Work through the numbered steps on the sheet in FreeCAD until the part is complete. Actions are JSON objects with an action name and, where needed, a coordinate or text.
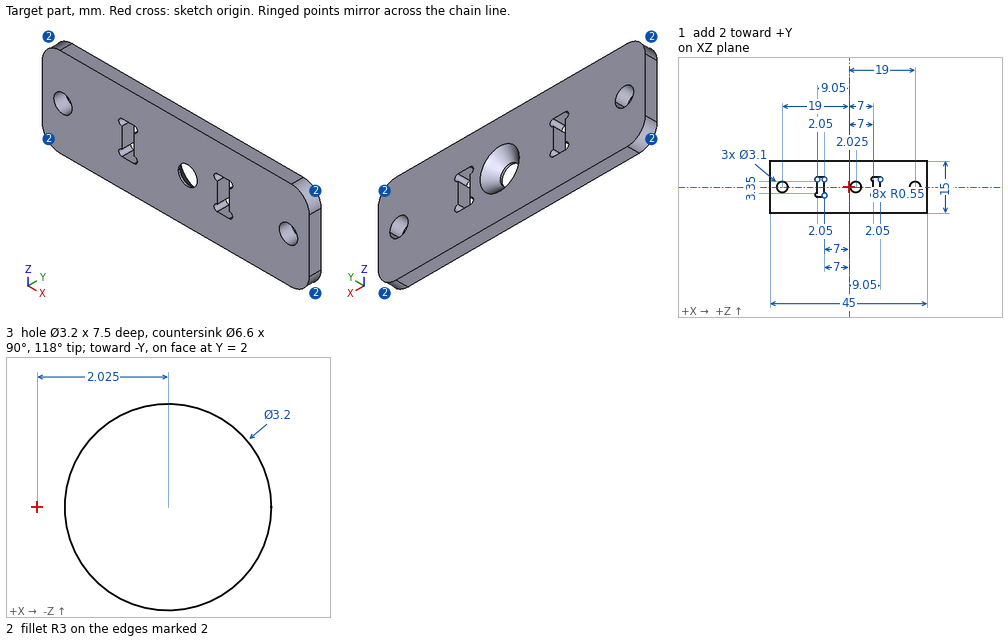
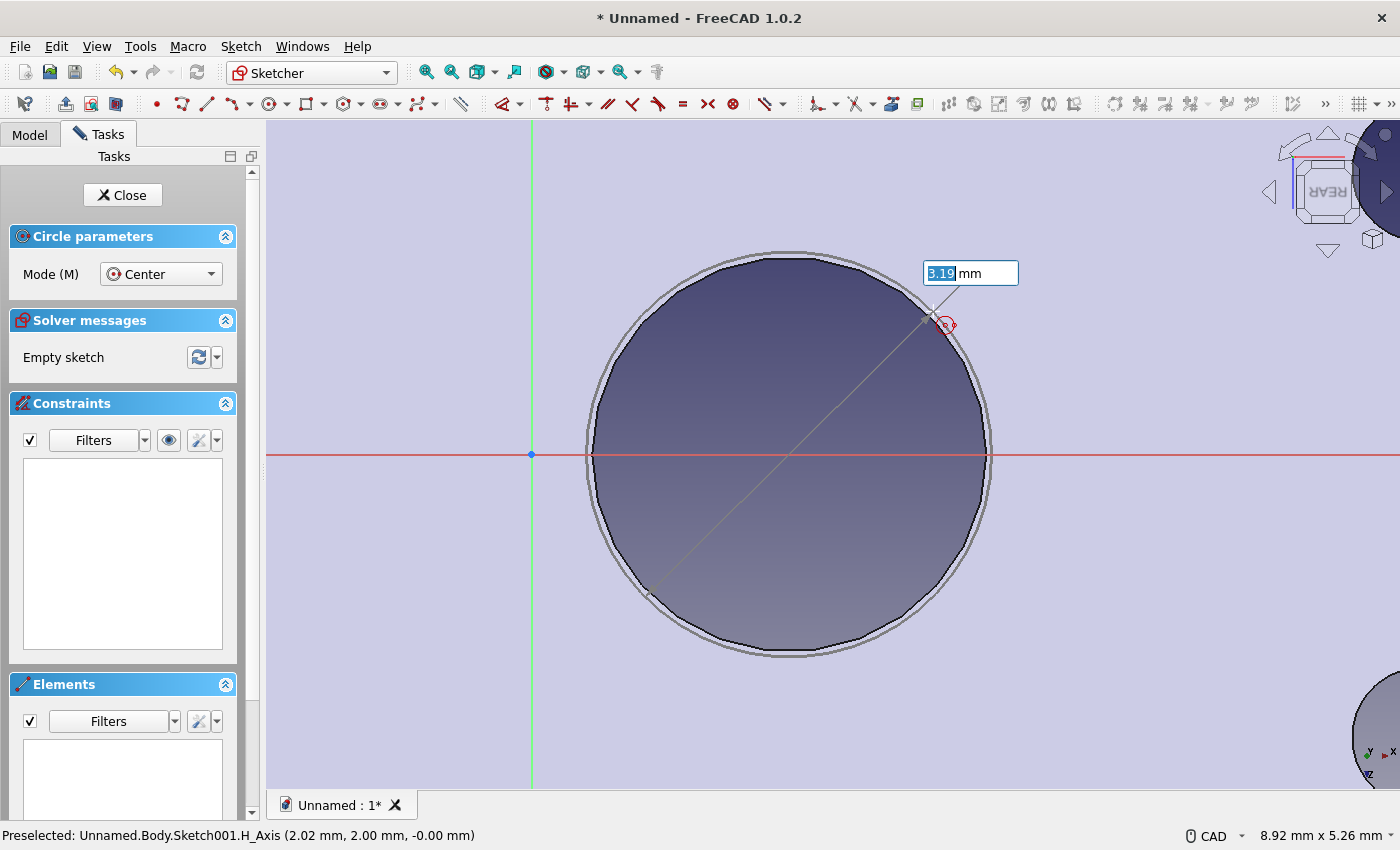
{"action": "type", "text": "3.2"}
{"action": "key", "text": "Return"}
{"action": "key", "text": "Escape"}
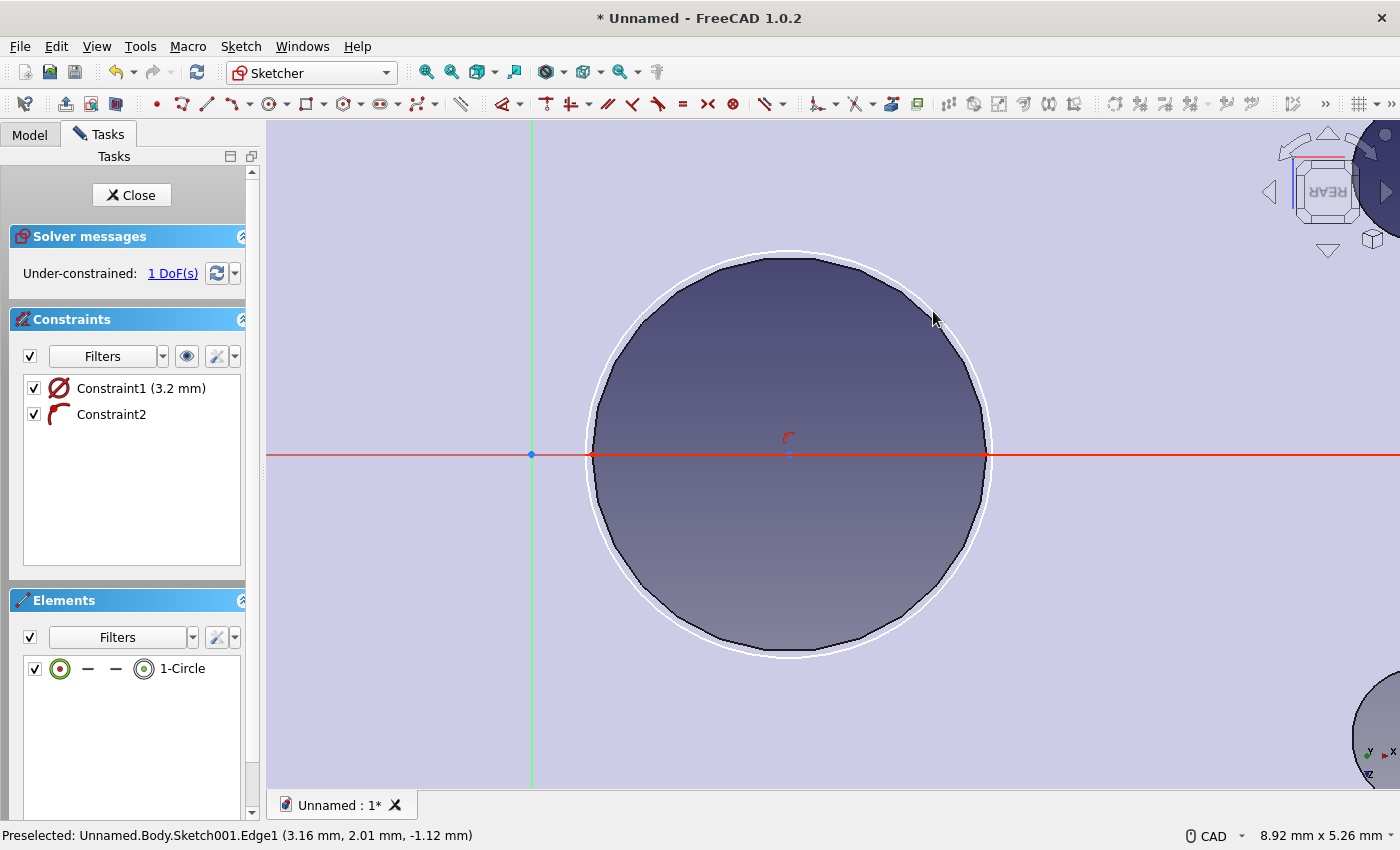
{"action": "left_click", "coordinate": [502, 104]}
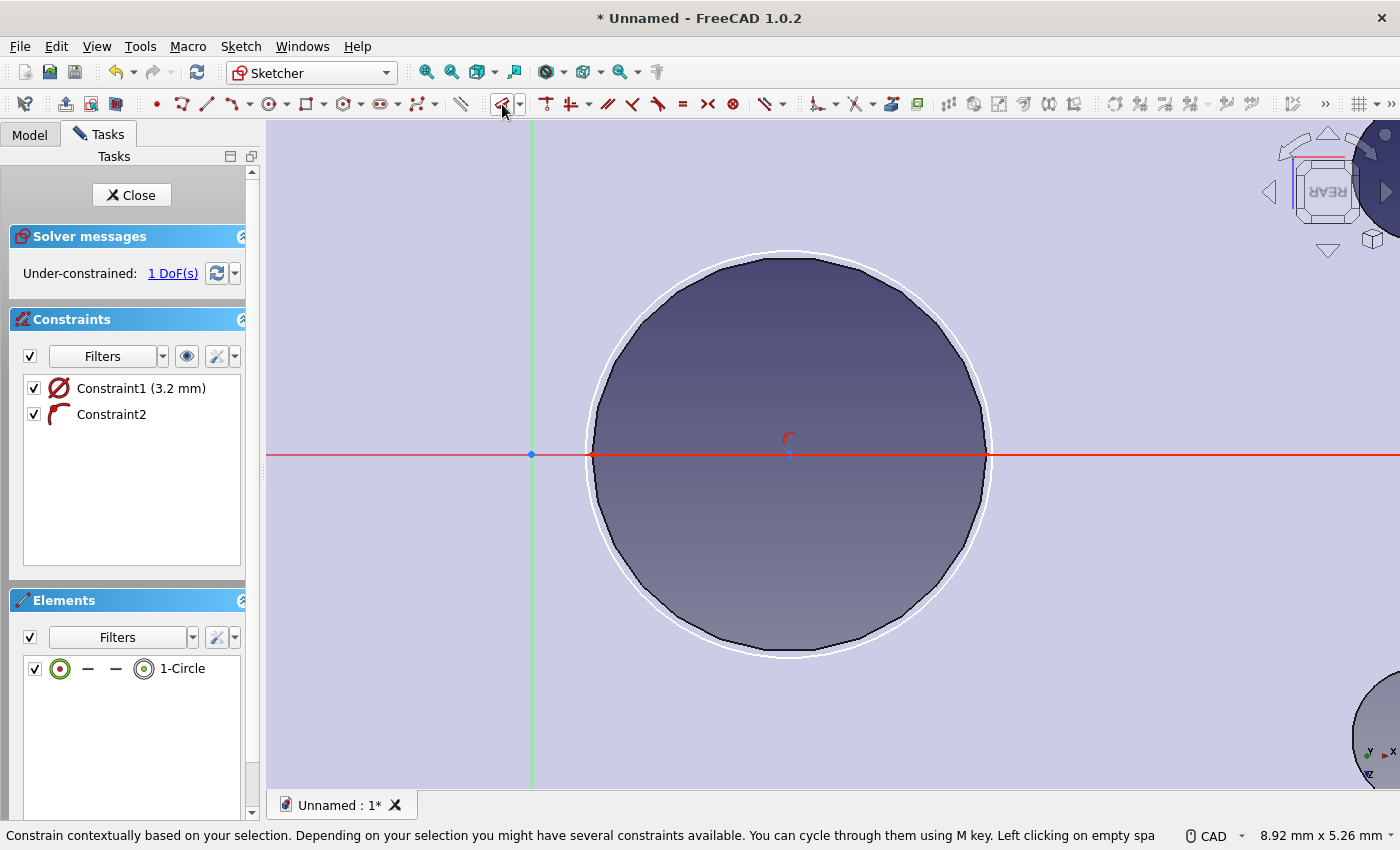
{"action": "left_click", "coordinate": [789, 454]}
{"action": "left_click", "coordinate": [660, 488]}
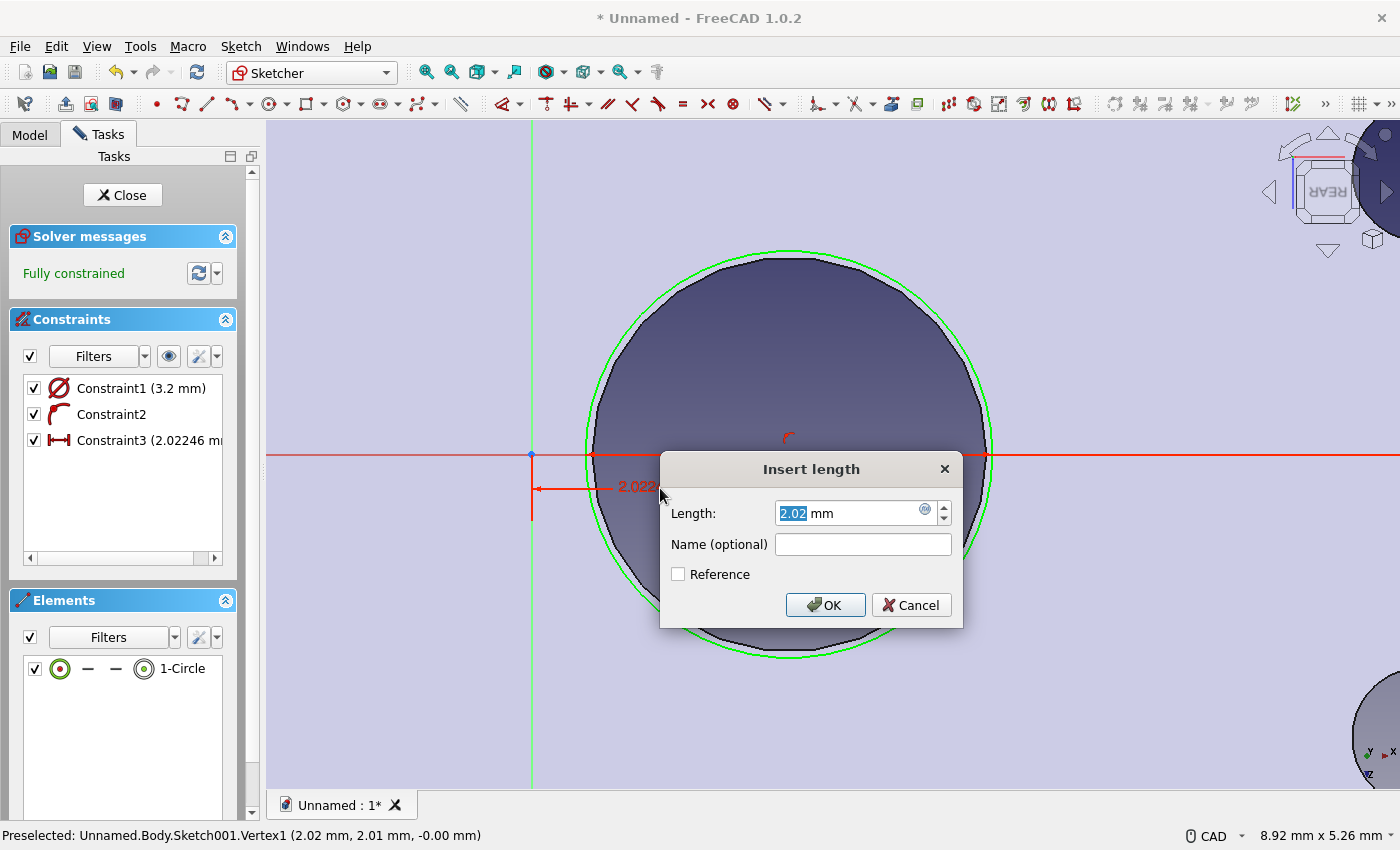
{"action": "type", "text": "2.025"}
{"action": "key", "text": "Return"}
{"action": "key", "text": "Escape"}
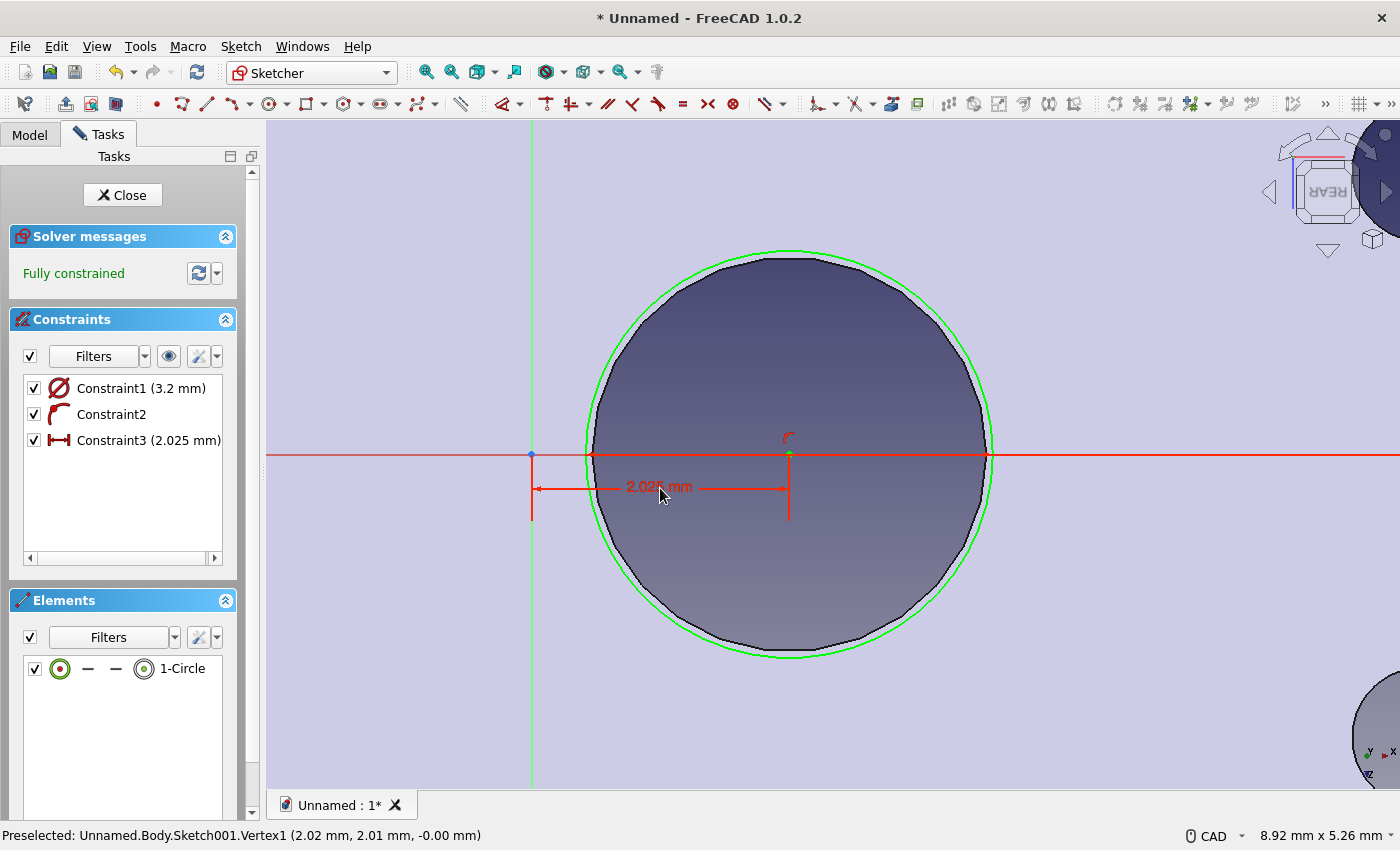
{"action": "left_click", "coordinate": [123, 195]}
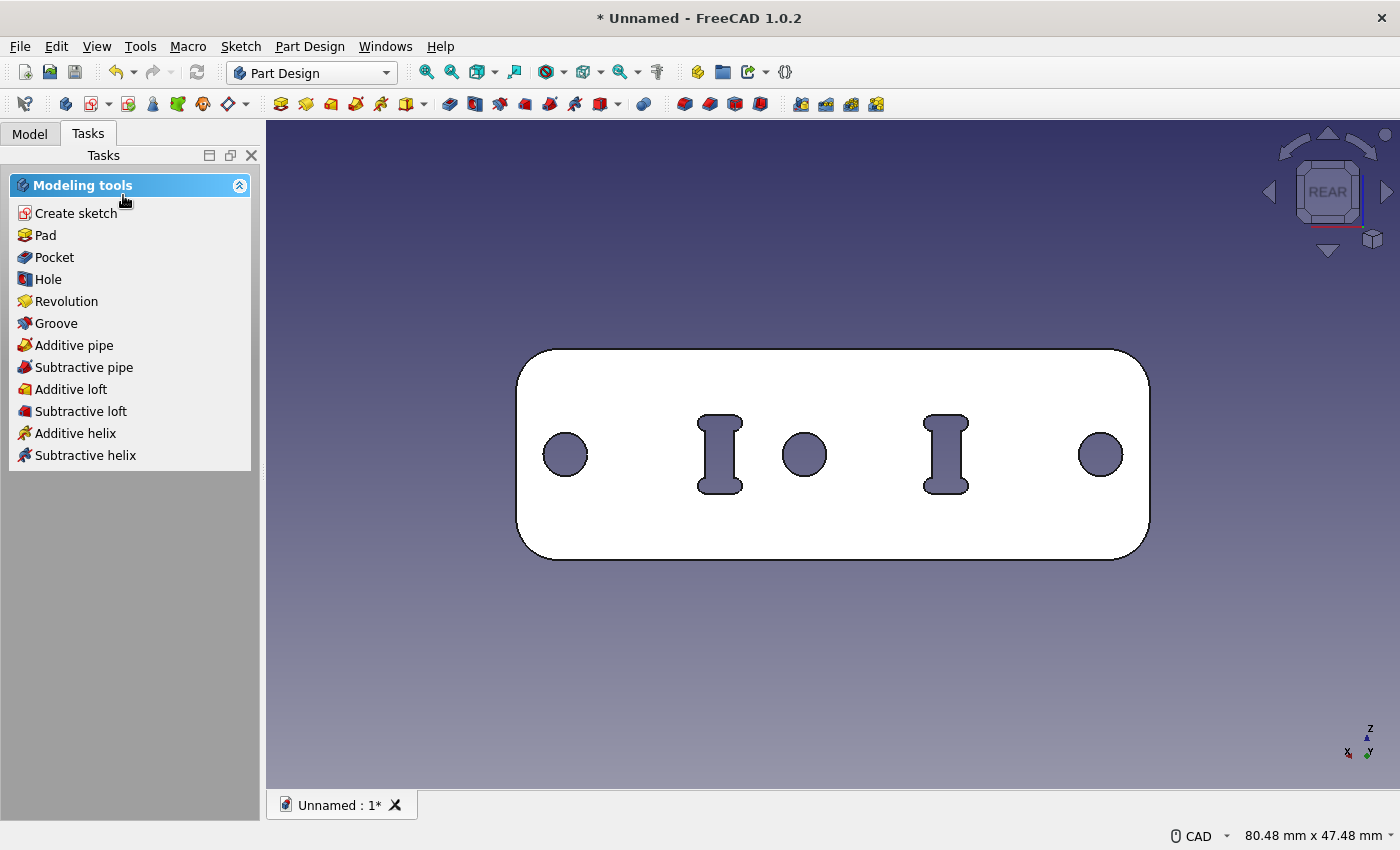
{"action": "left_click", "coordinate": [475, 104]}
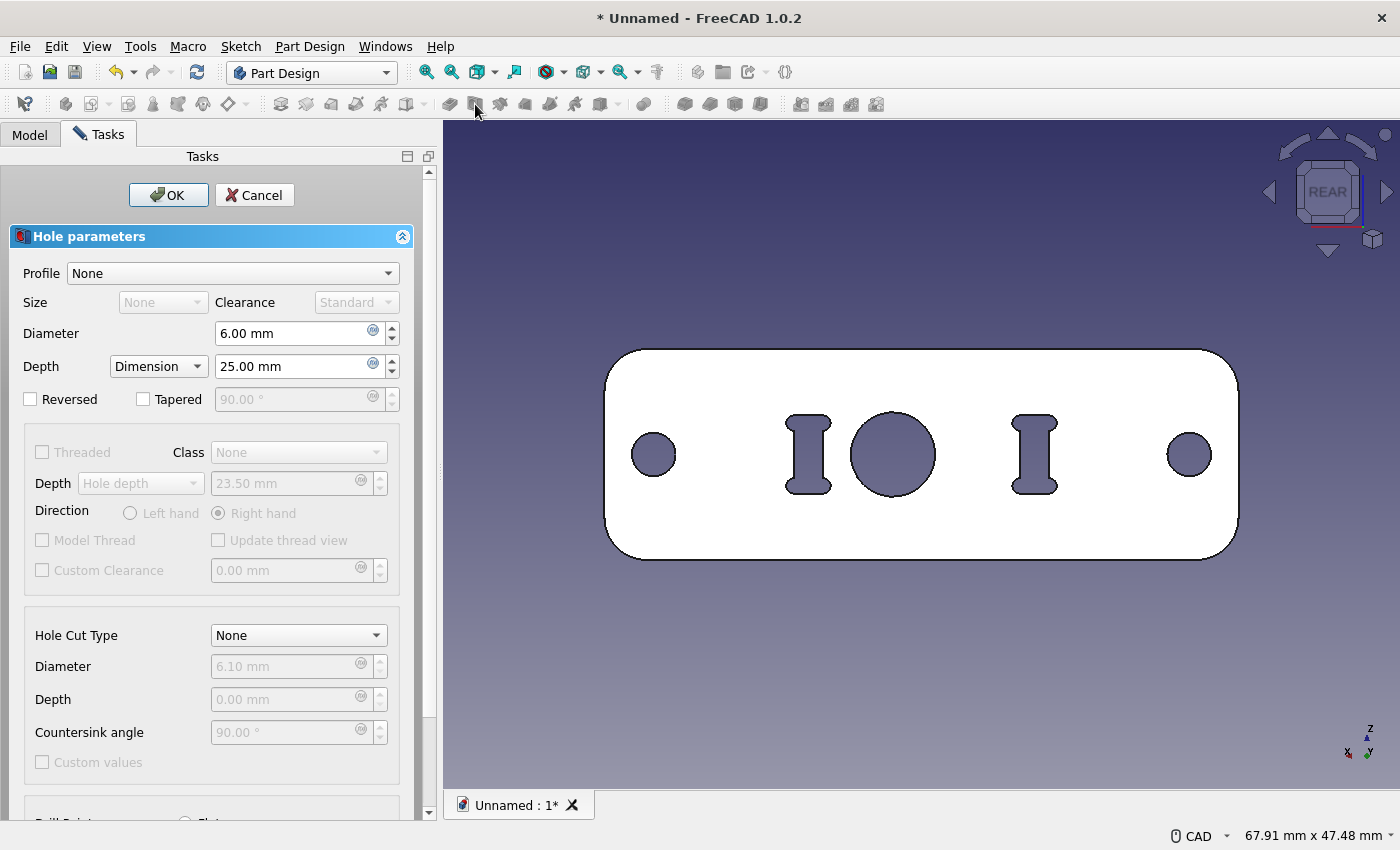
{"action": "triple_click", "coordinate": [300, 334]}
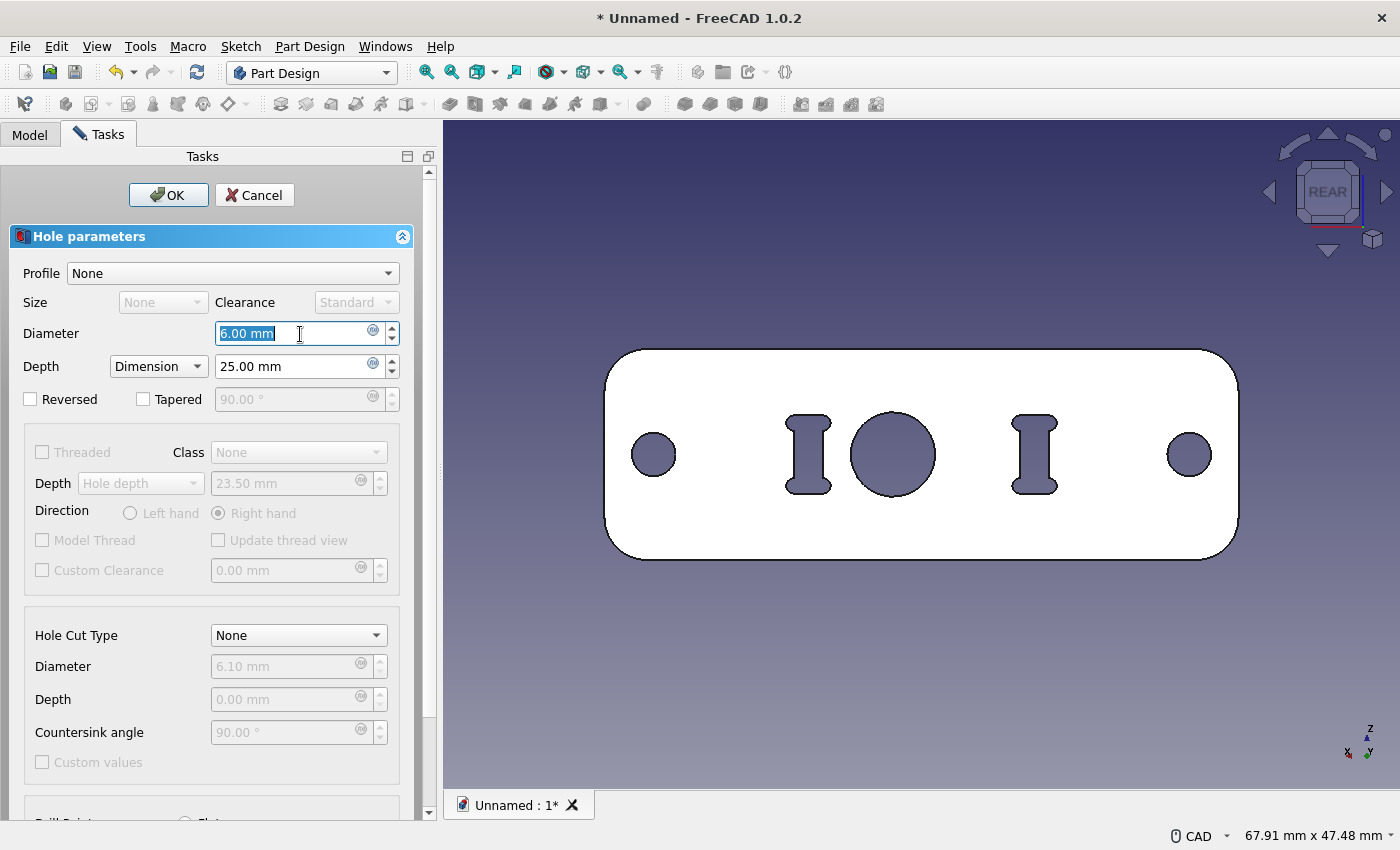
{"action": "type", "text": "3.2"}
{"action": "key", "text": "Tab"}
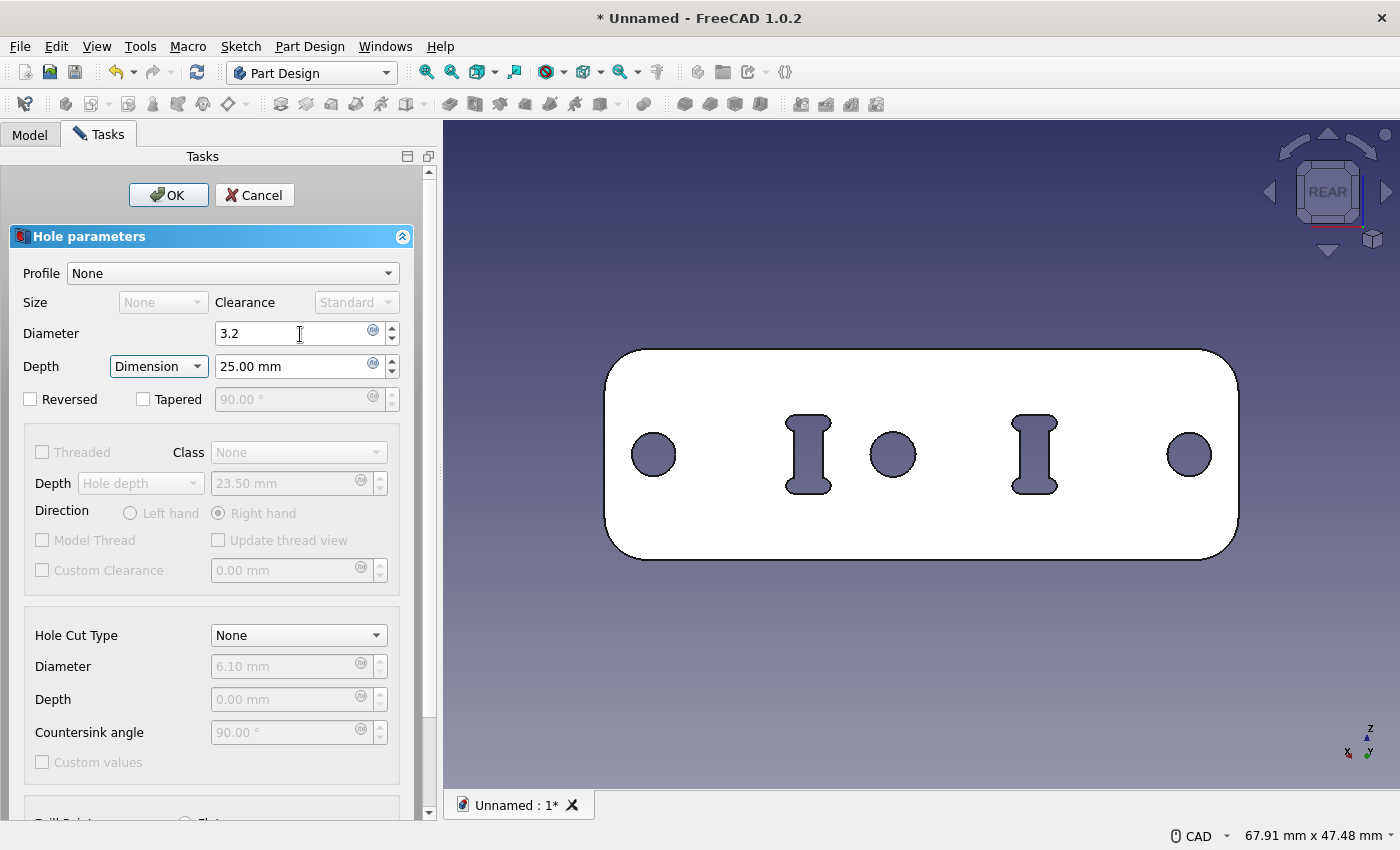
{"action": "triple_click", "coordinate": [300, 366]}